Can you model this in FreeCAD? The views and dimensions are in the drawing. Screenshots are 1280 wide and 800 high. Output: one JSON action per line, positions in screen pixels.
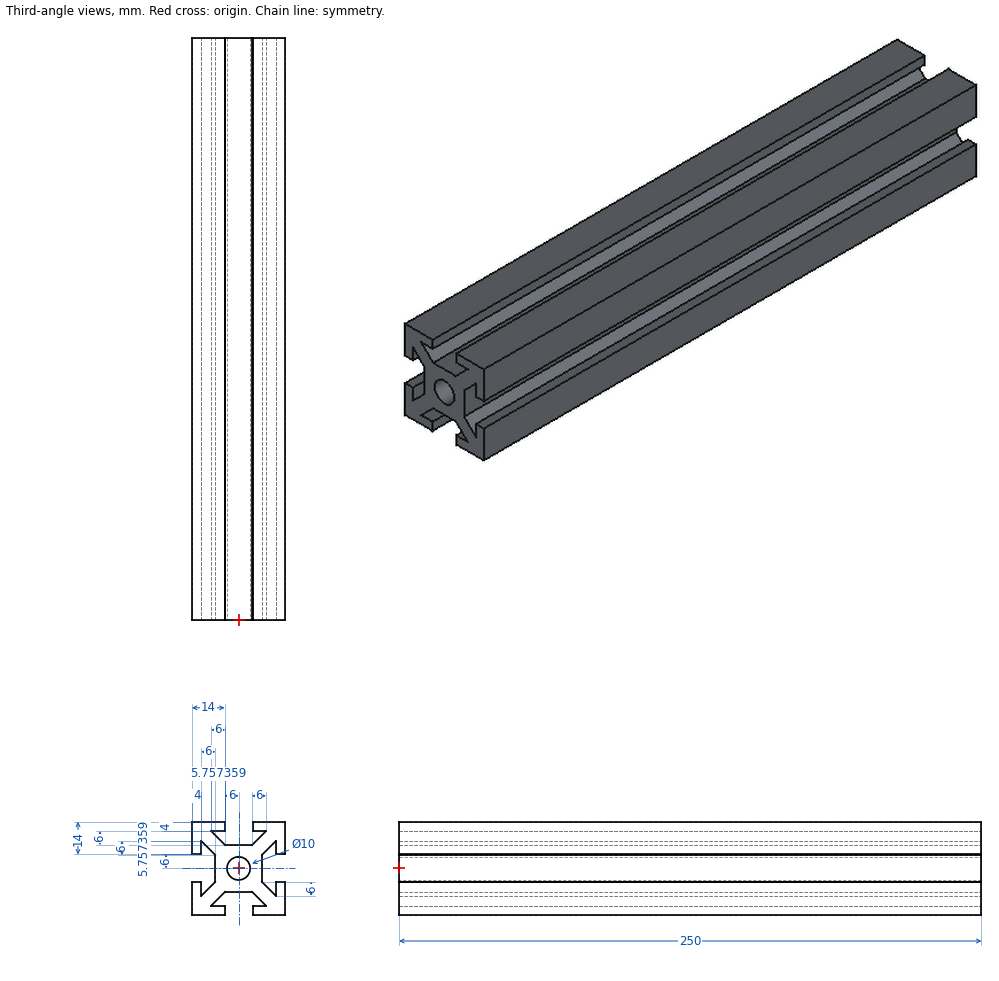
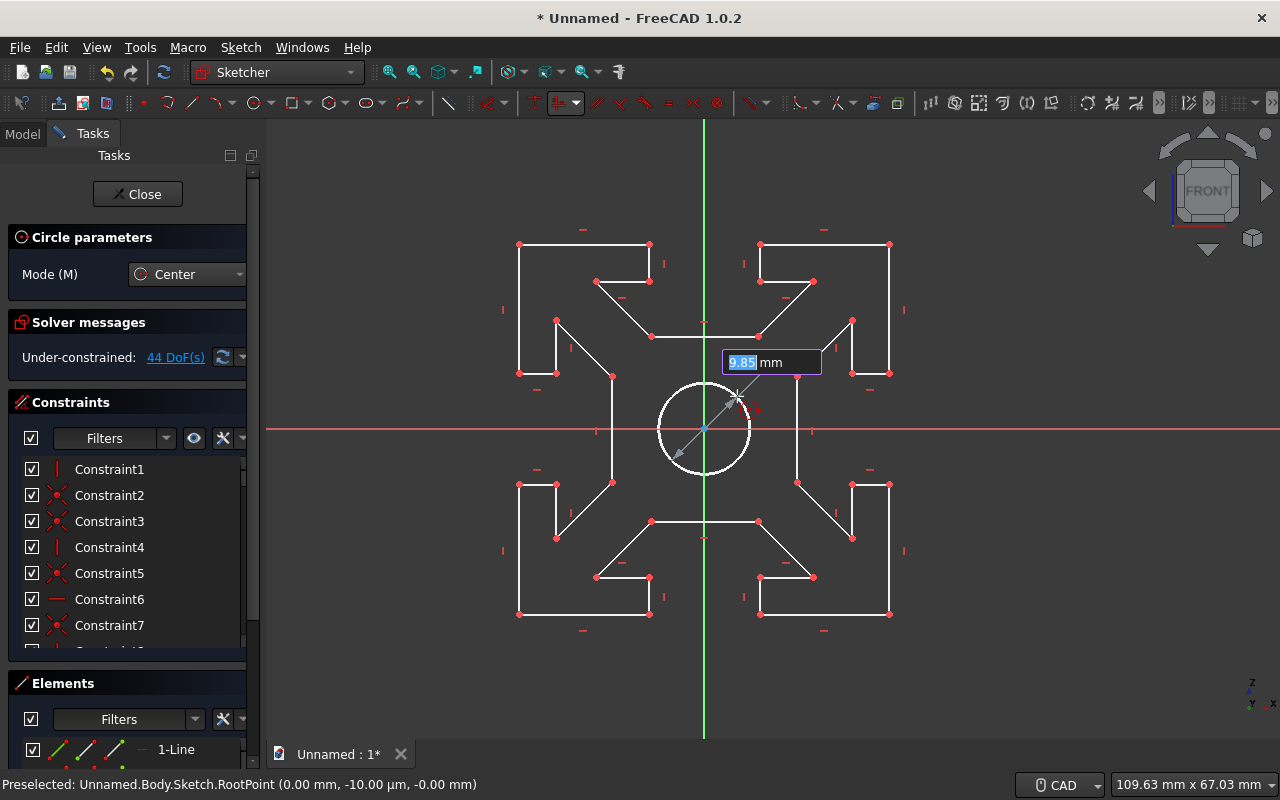
{"action": "type", "text": "10"}
{"action": "key", "text": "Return"}
{"action": "key", "text": "Escape"}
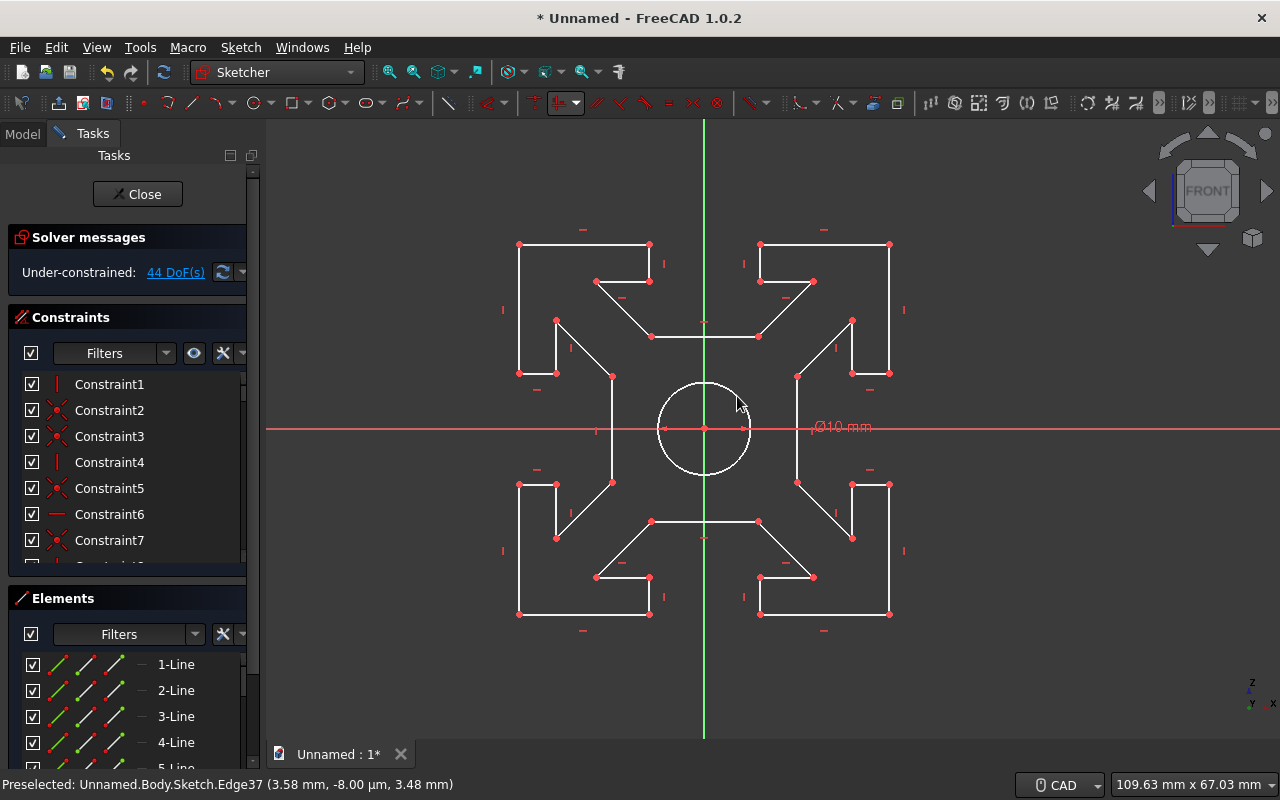
{"action": "left_click", "coordinate": [596, 282]}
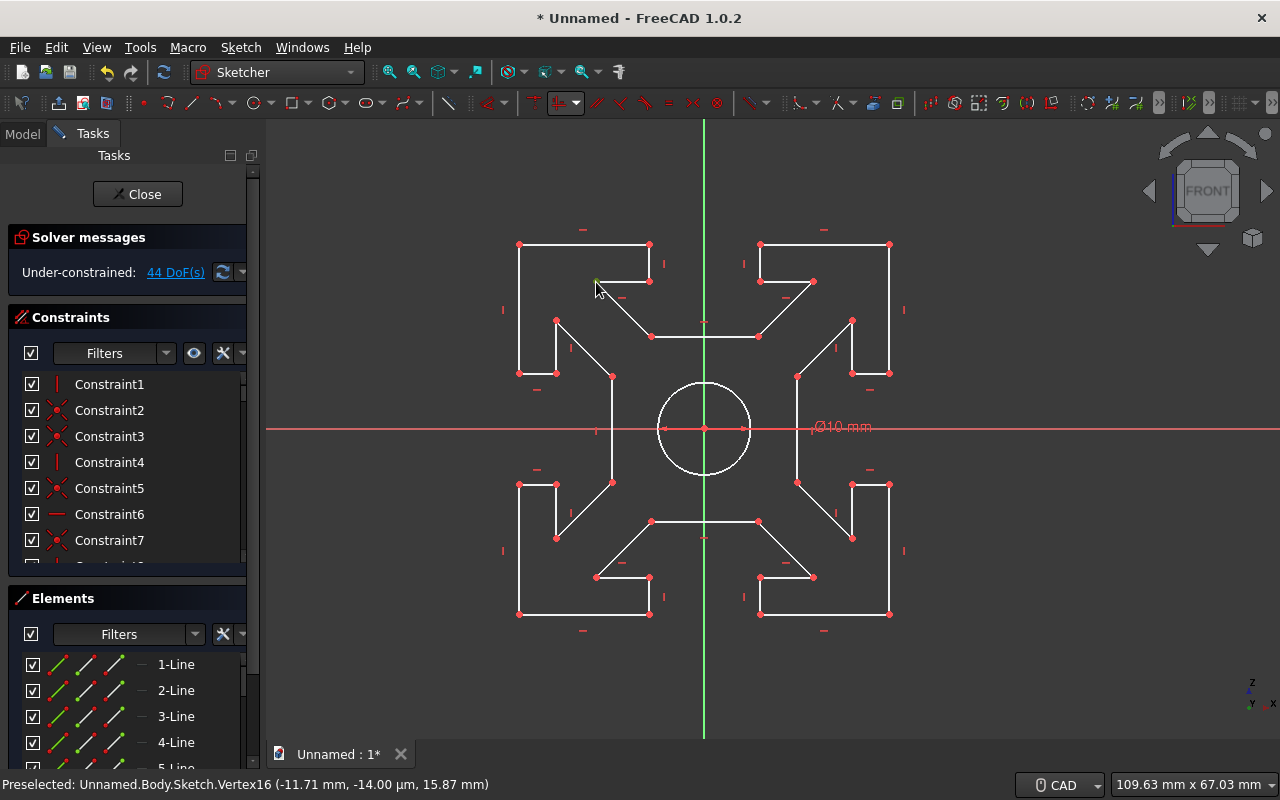
{"action": "left_click", "coordinate": [813, 282]}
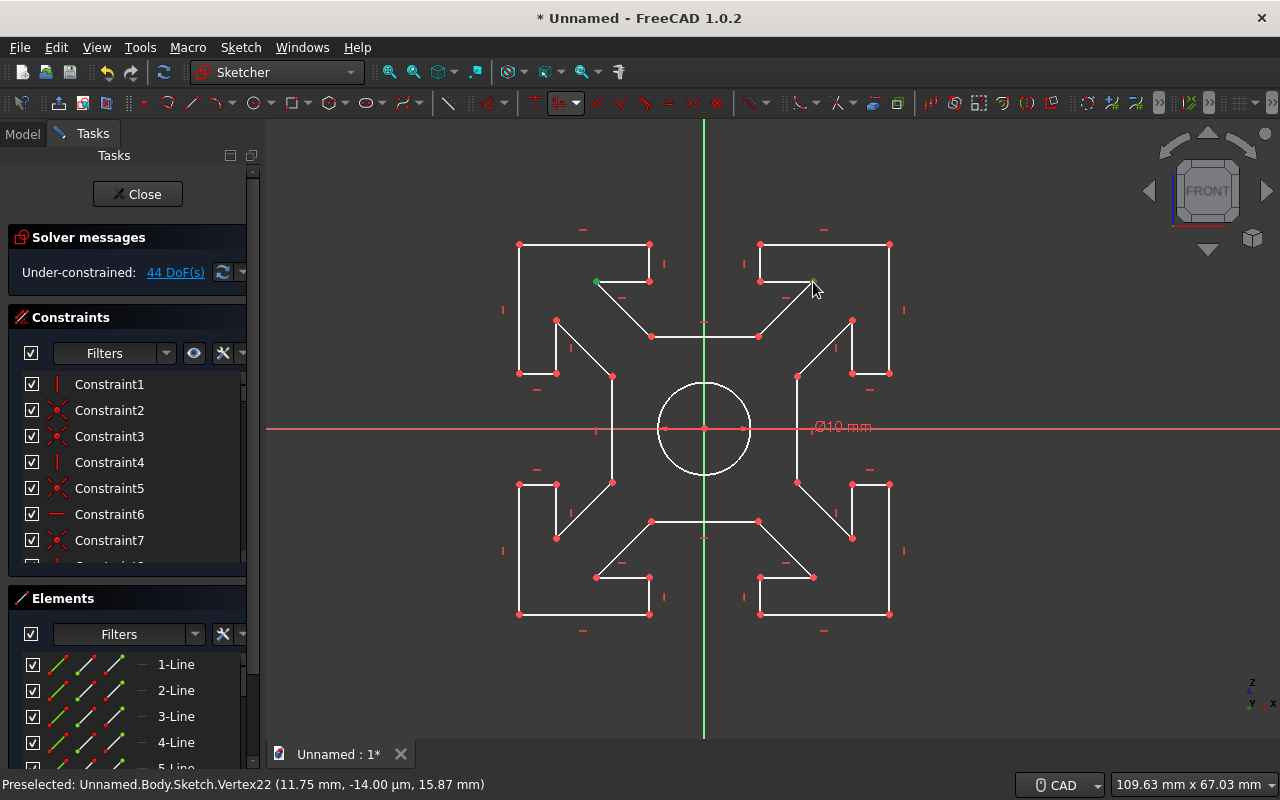
{"action": "left_click", "coordinate": [704, 671]}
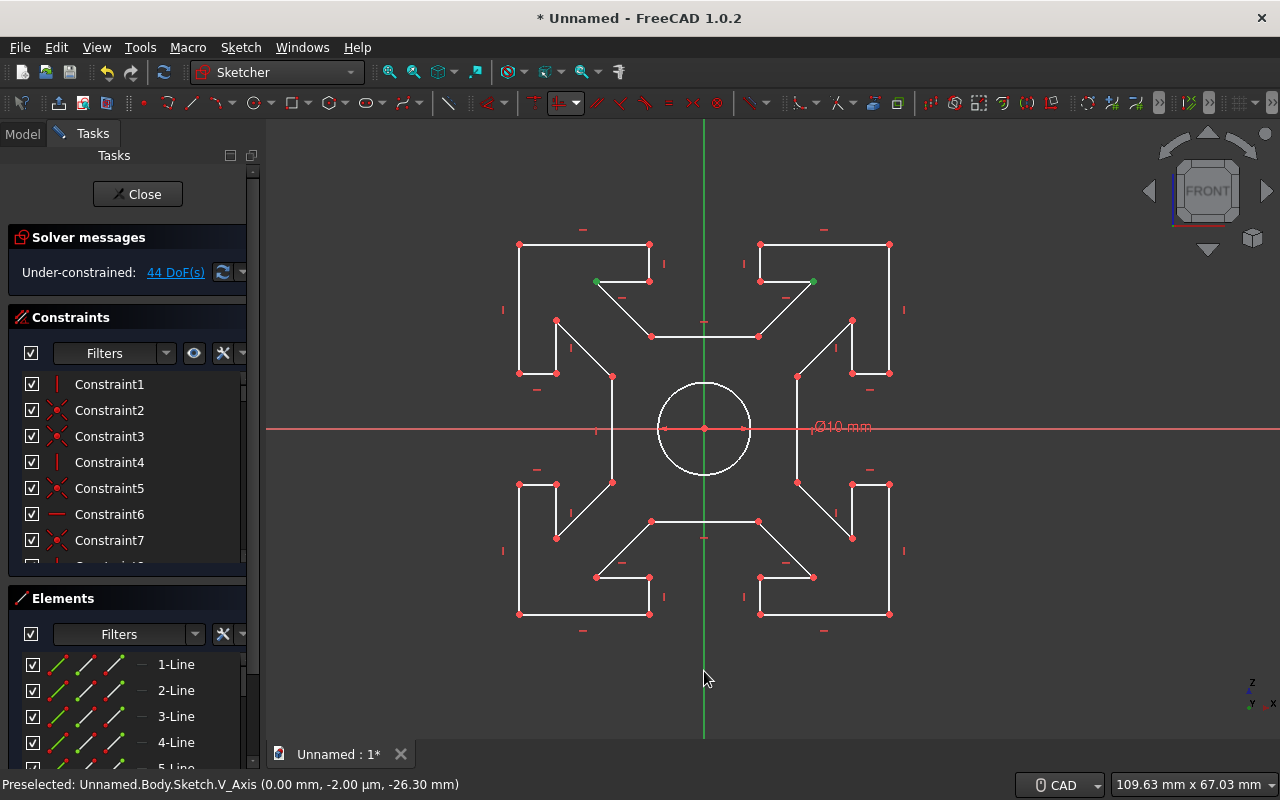
{"action": "left_click", "coordinate": [694, 104]}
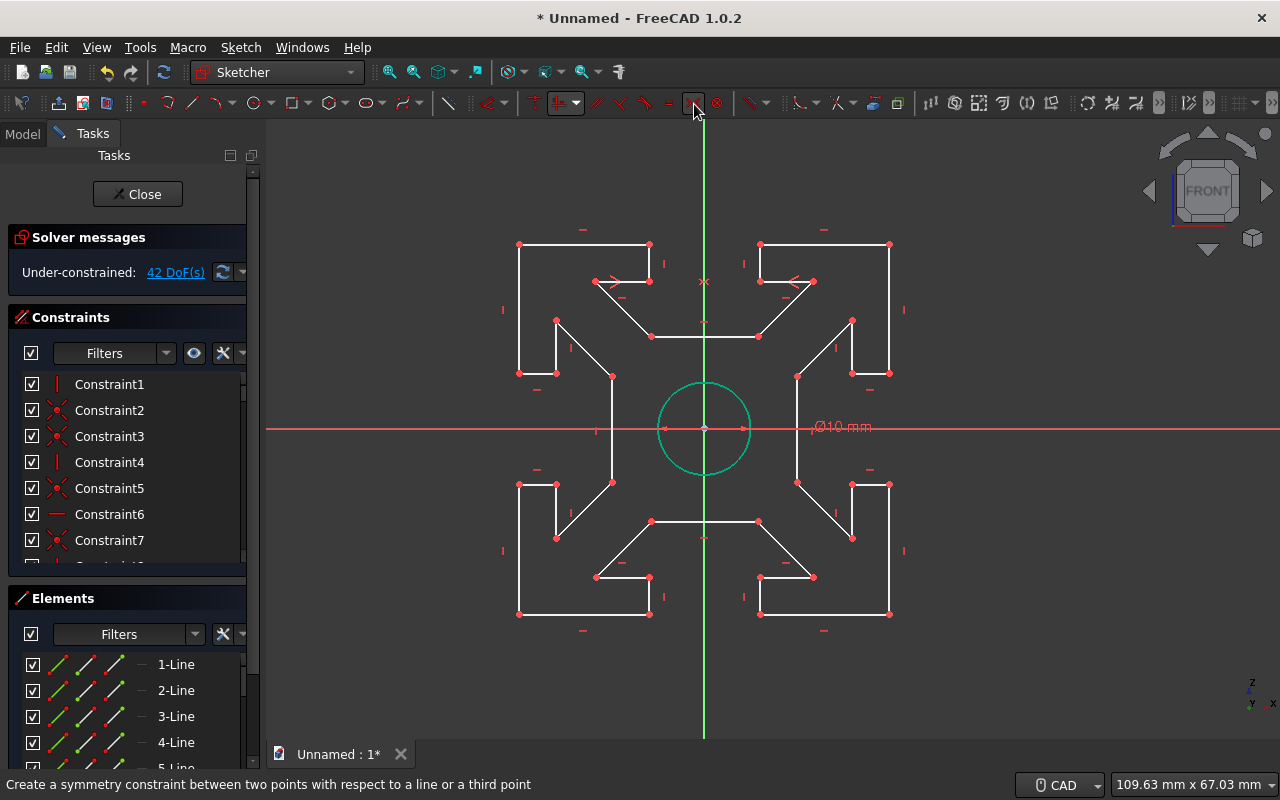
{"action": "left_click", "coordinate": [649, 245]}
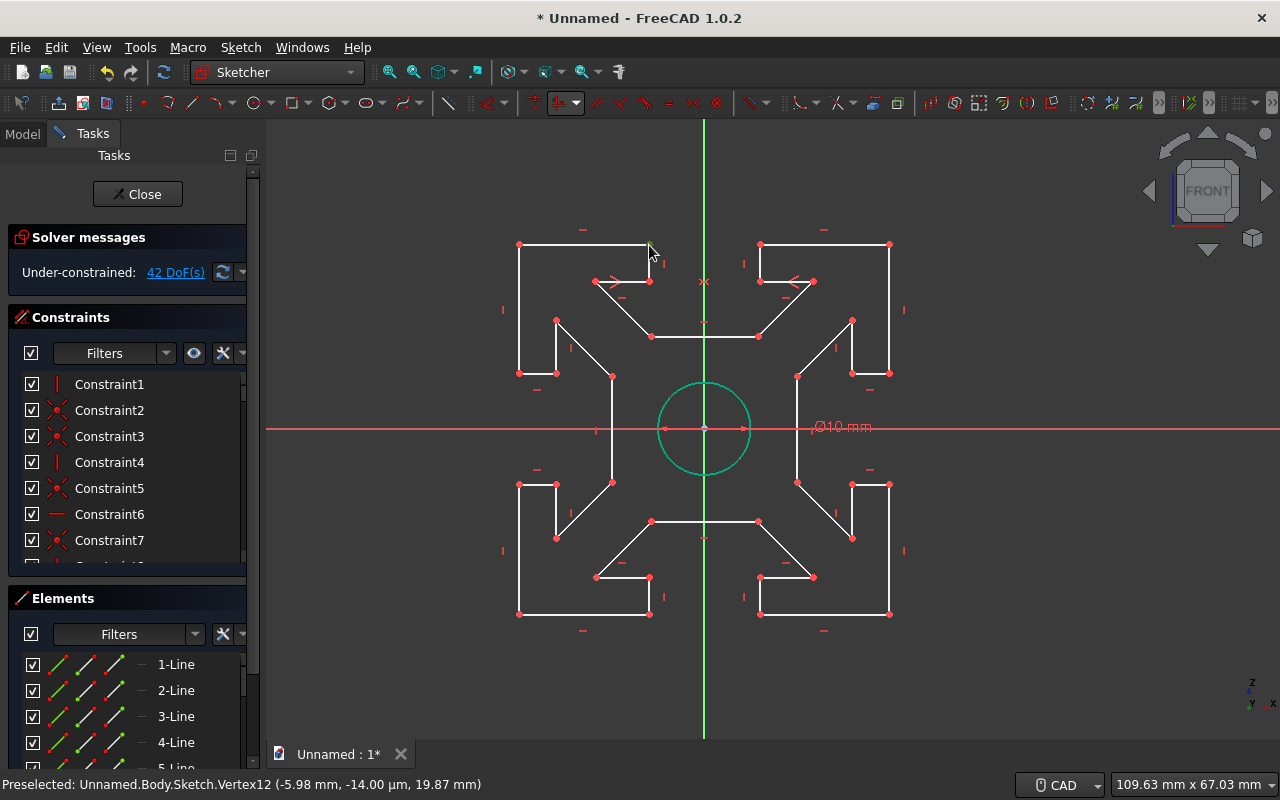
{"action": "left_click", "coordinate": [760, 245]}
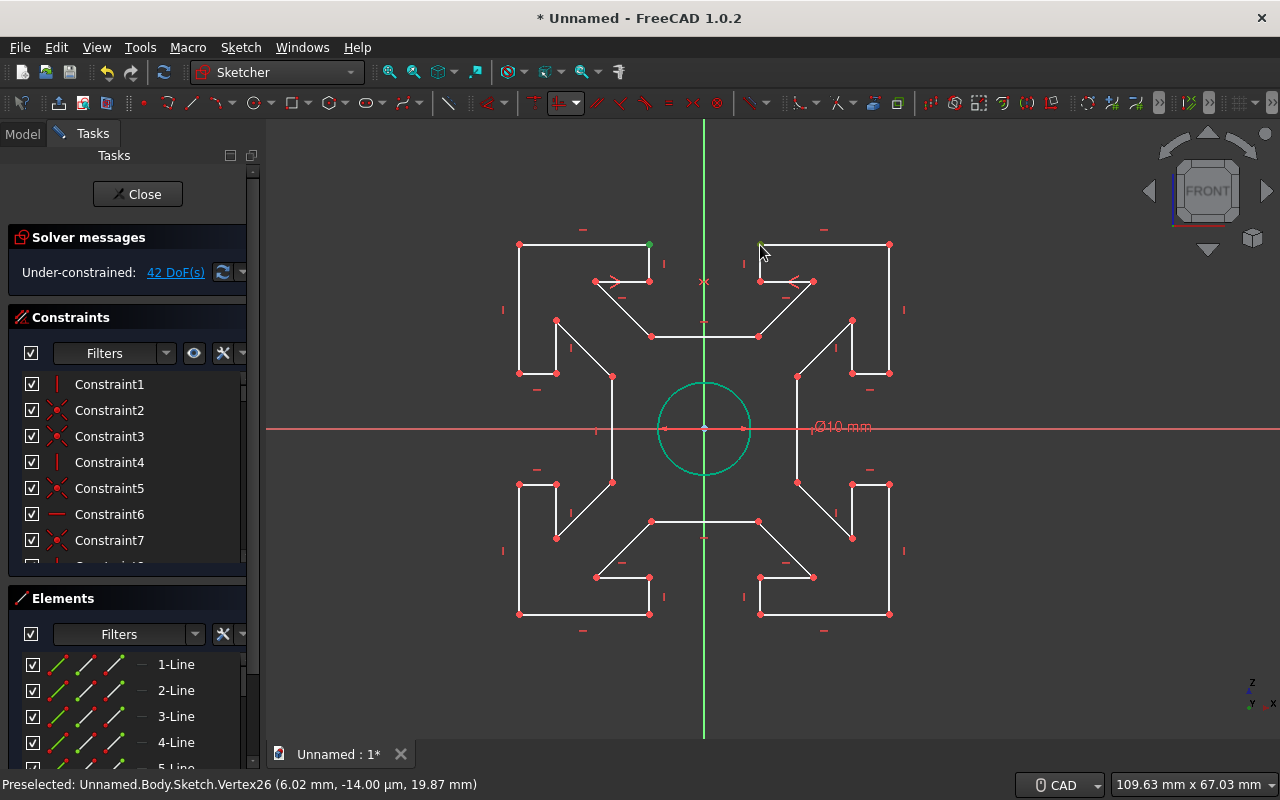
{"action": "left_click", "coordinate": [704, 671]}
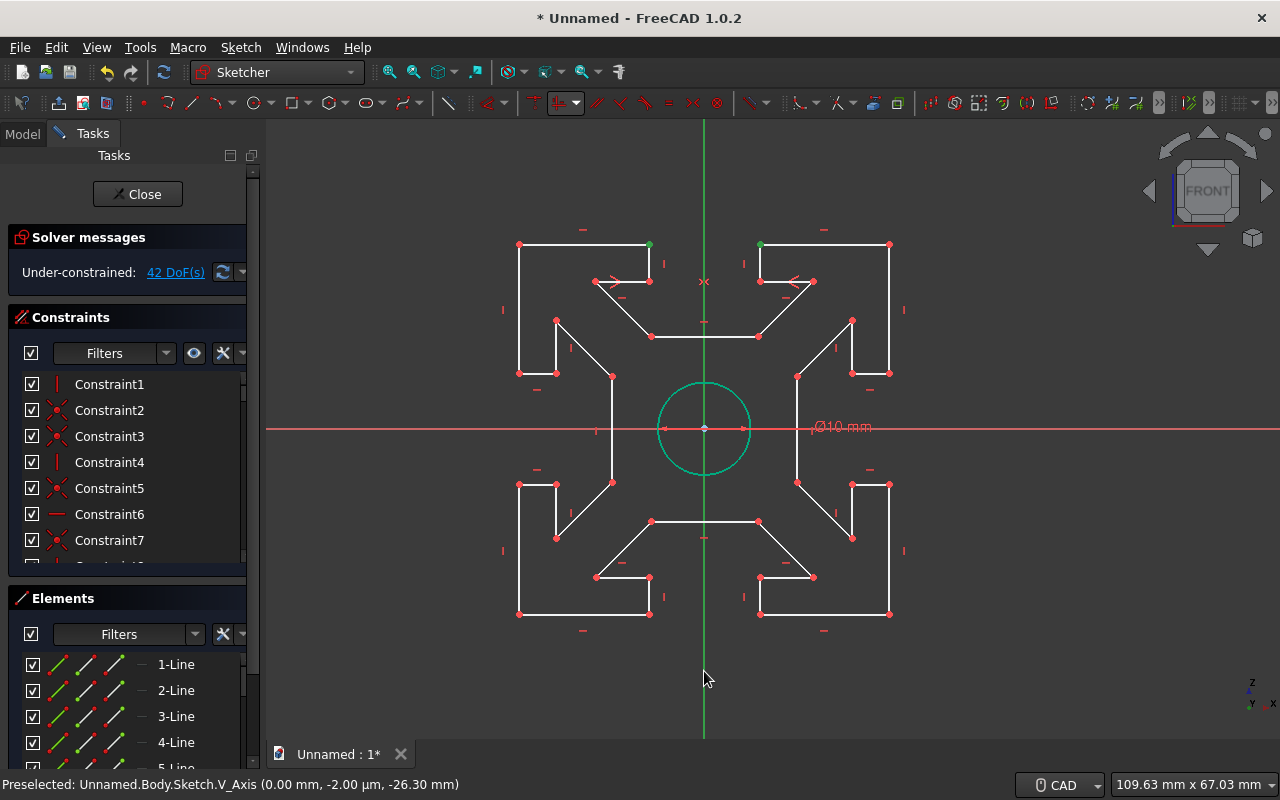
{"action": "left_click", "coordinate": [694, 104]}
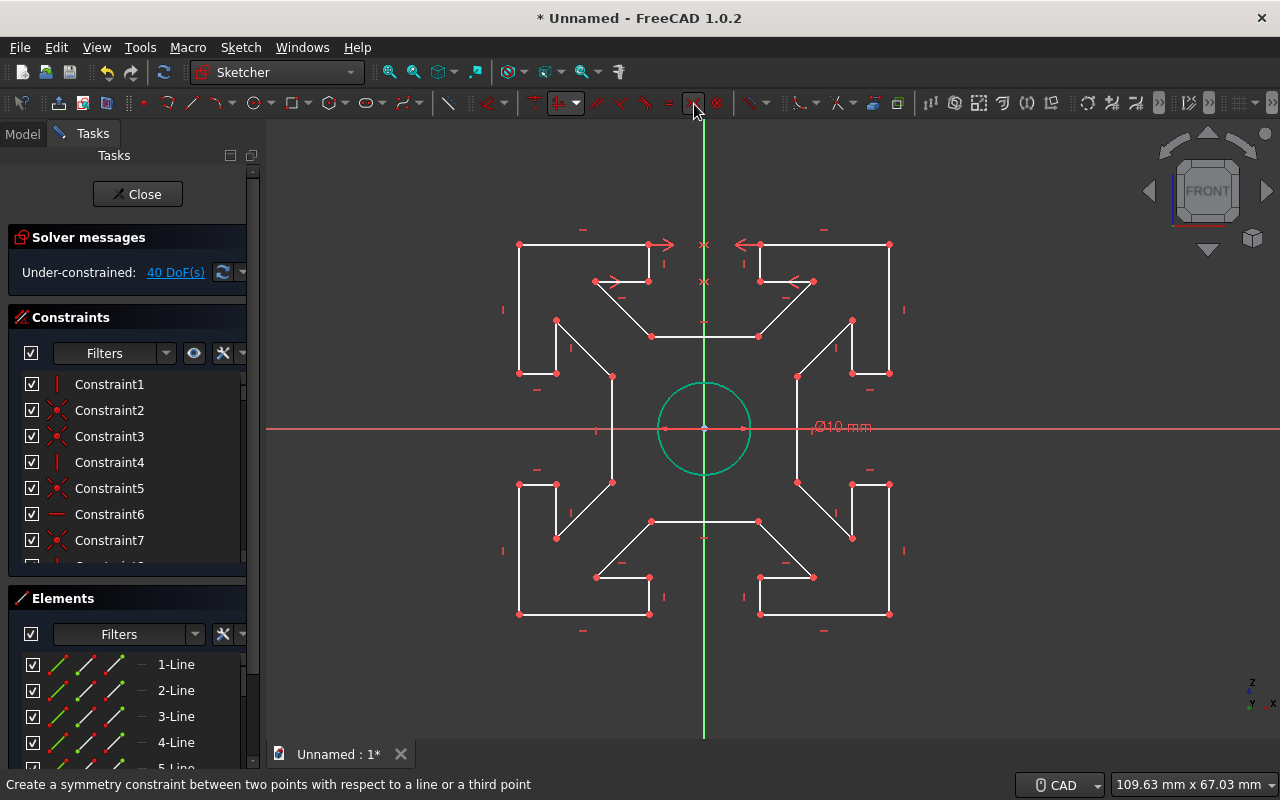
{"action": "left_click", "coordinate": [519, 374]}